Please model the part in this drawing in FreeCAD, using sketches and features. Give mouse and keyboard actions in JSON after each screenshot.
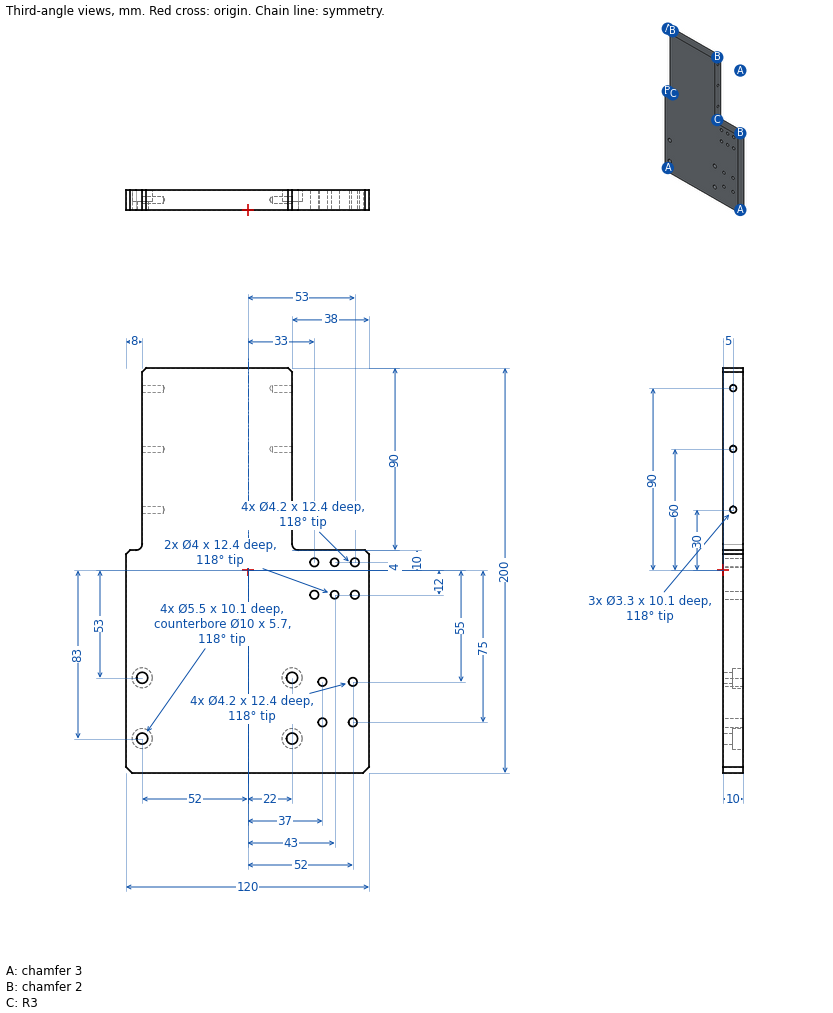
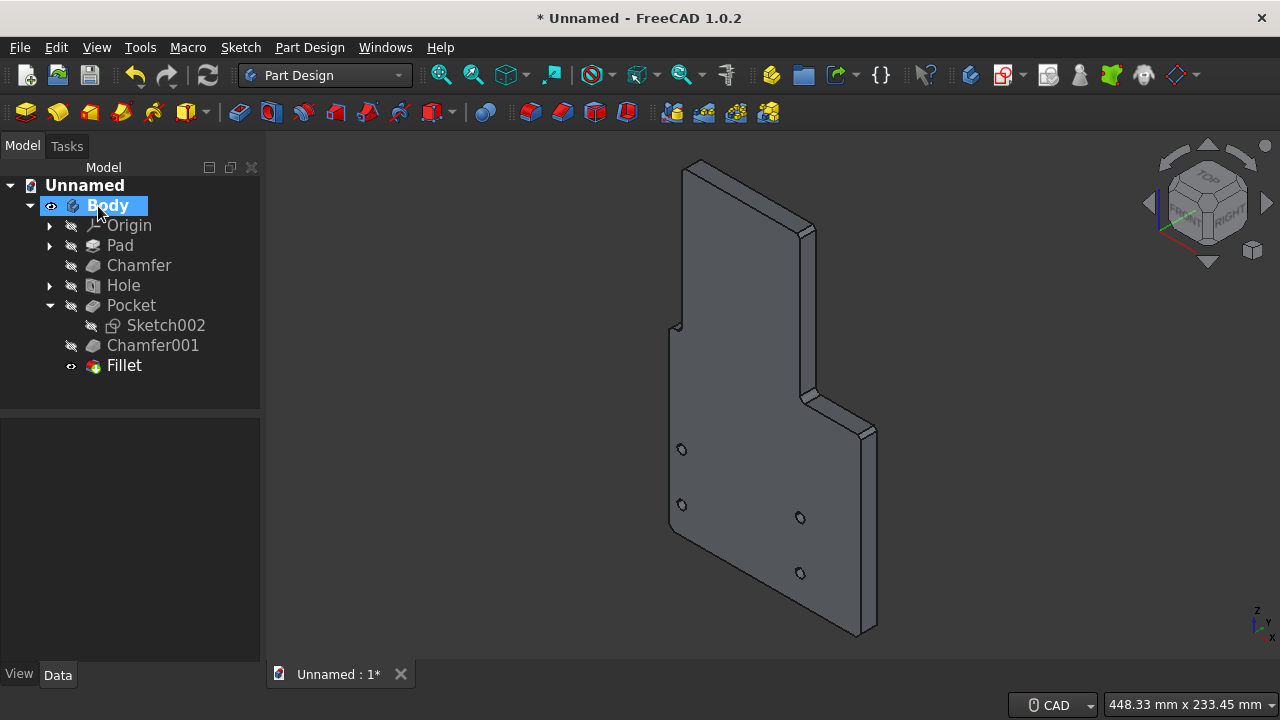
{"action": "key", "text": "6"}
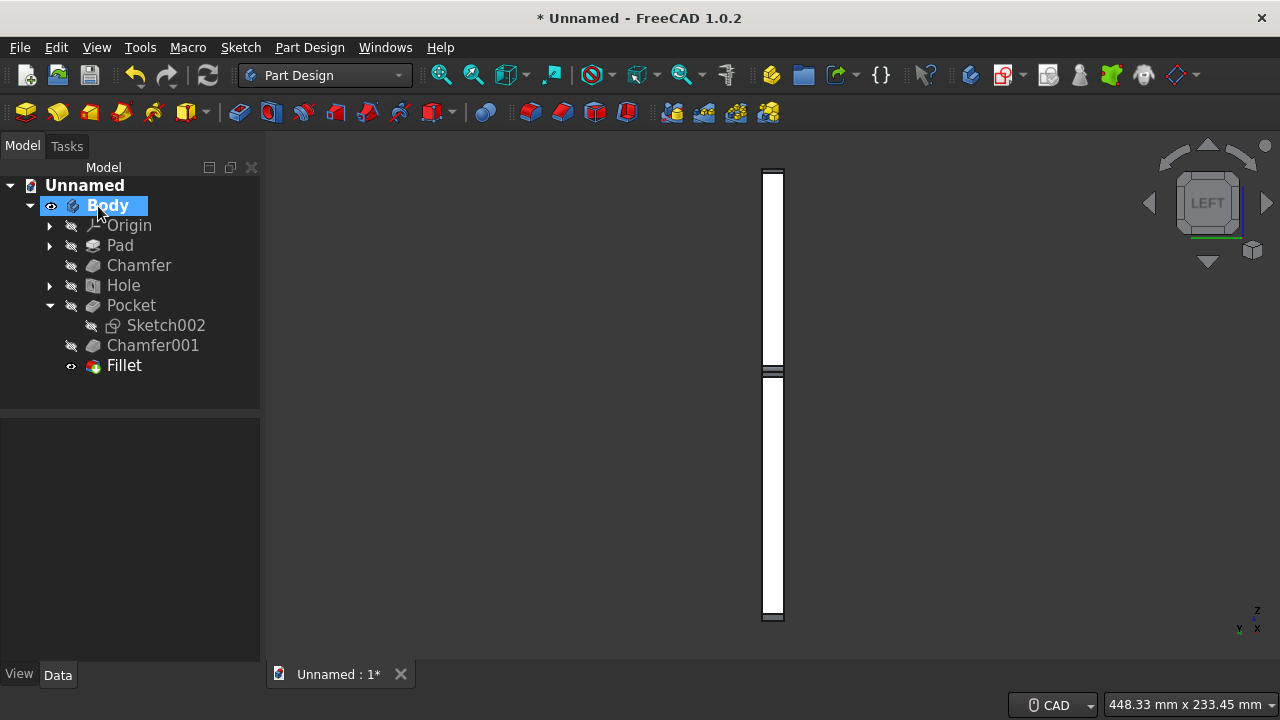
{"action": "left_click", "coordinate": [773, 323]}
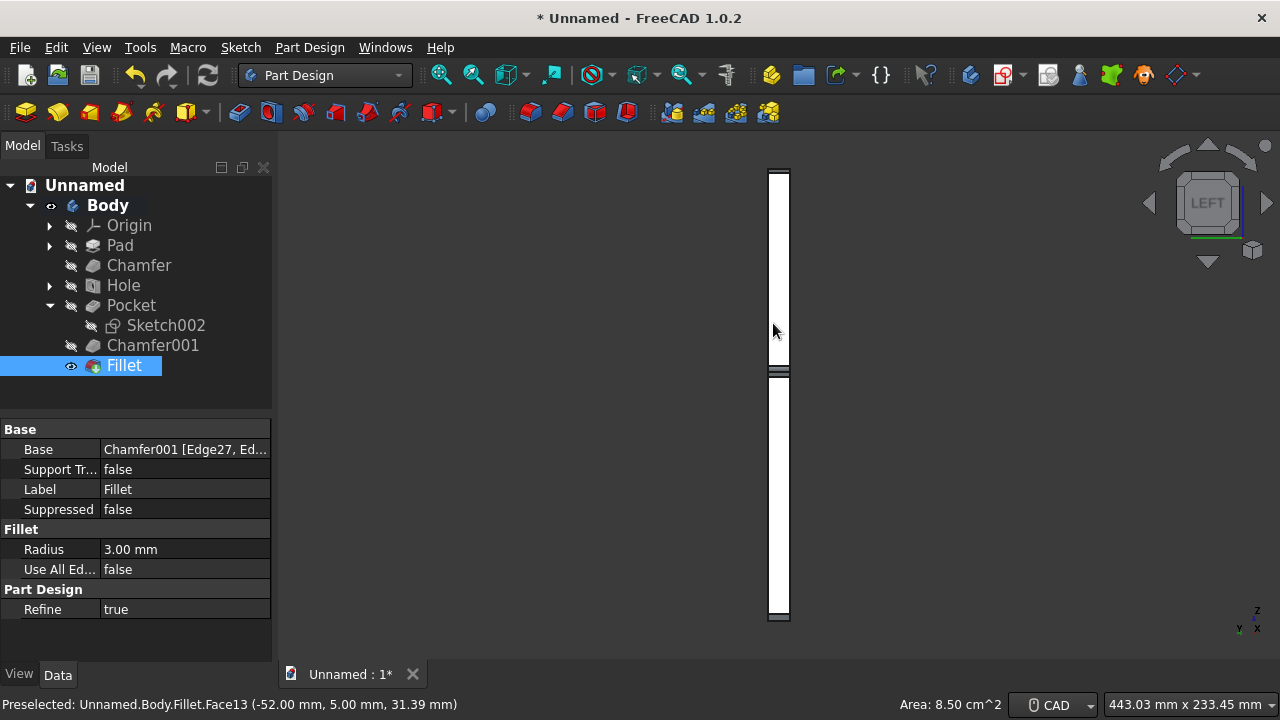
{"action": "left_click", "coordinate": [1004, 76]}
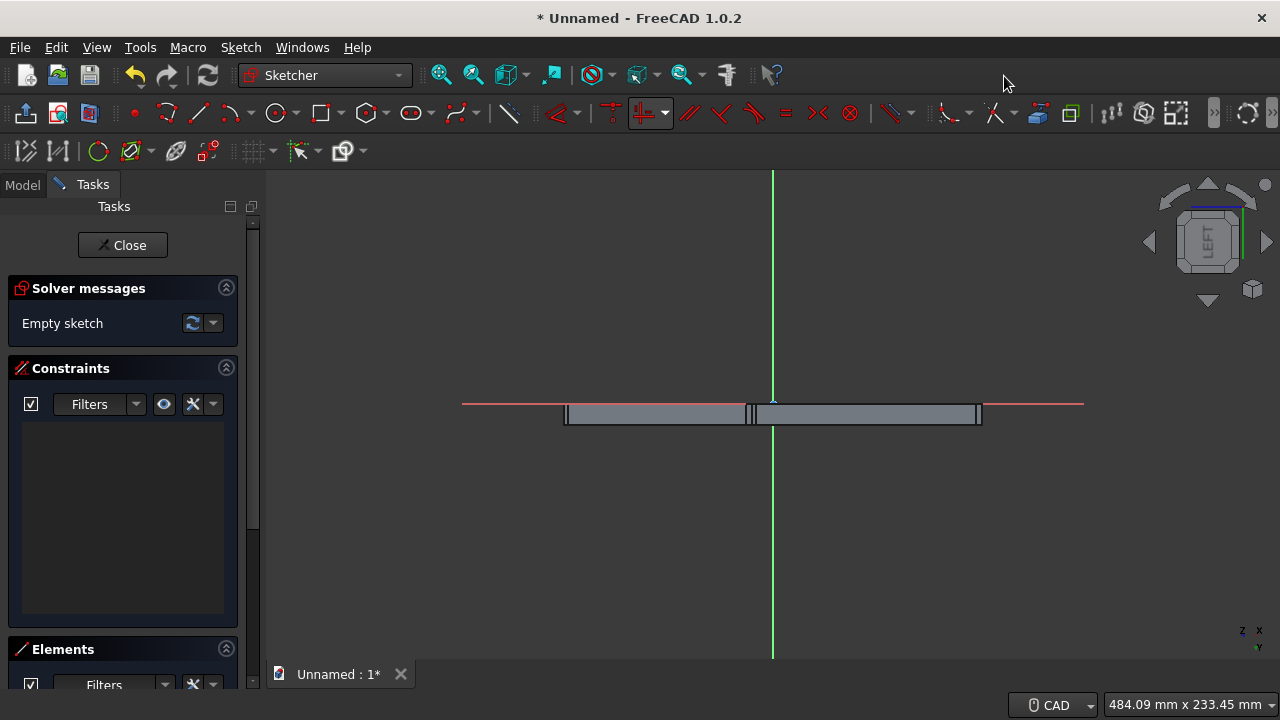
{"action": "left_click", "coordinate": [90, 114]}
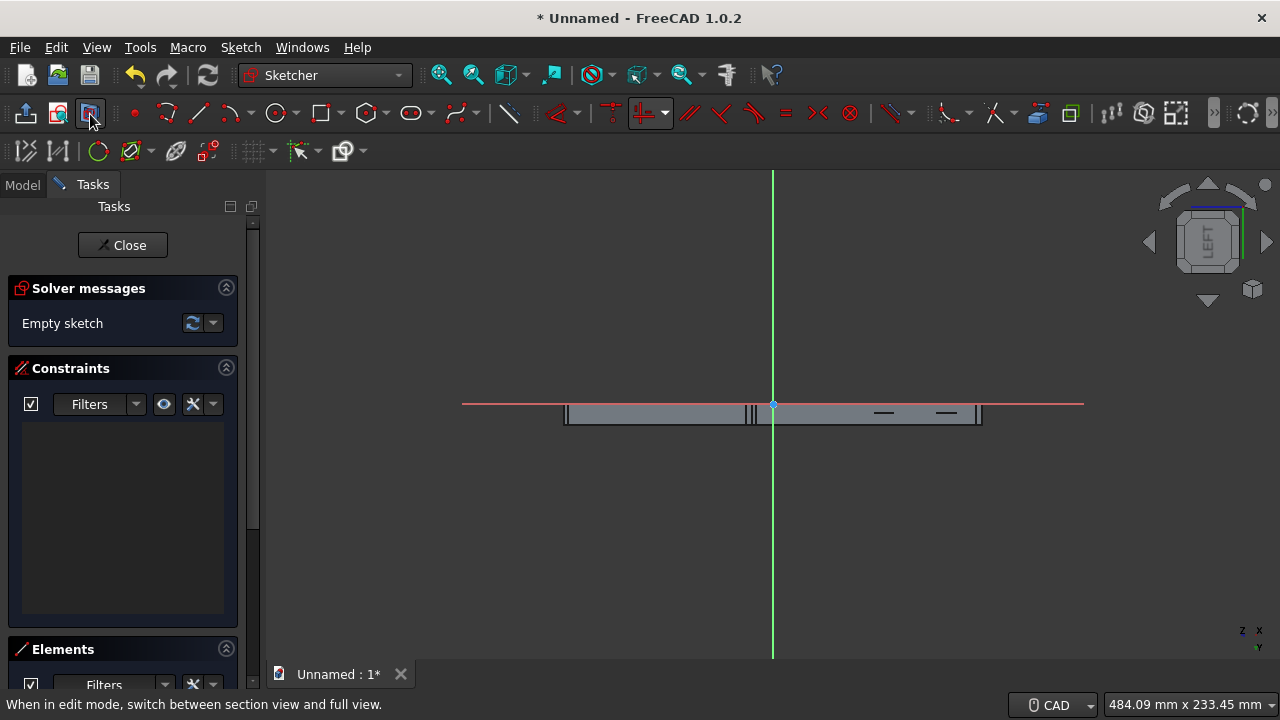
{"action": "scroll", "coordinate": [665, 409], "scroll_direction": "up", "scroll_amount": 6}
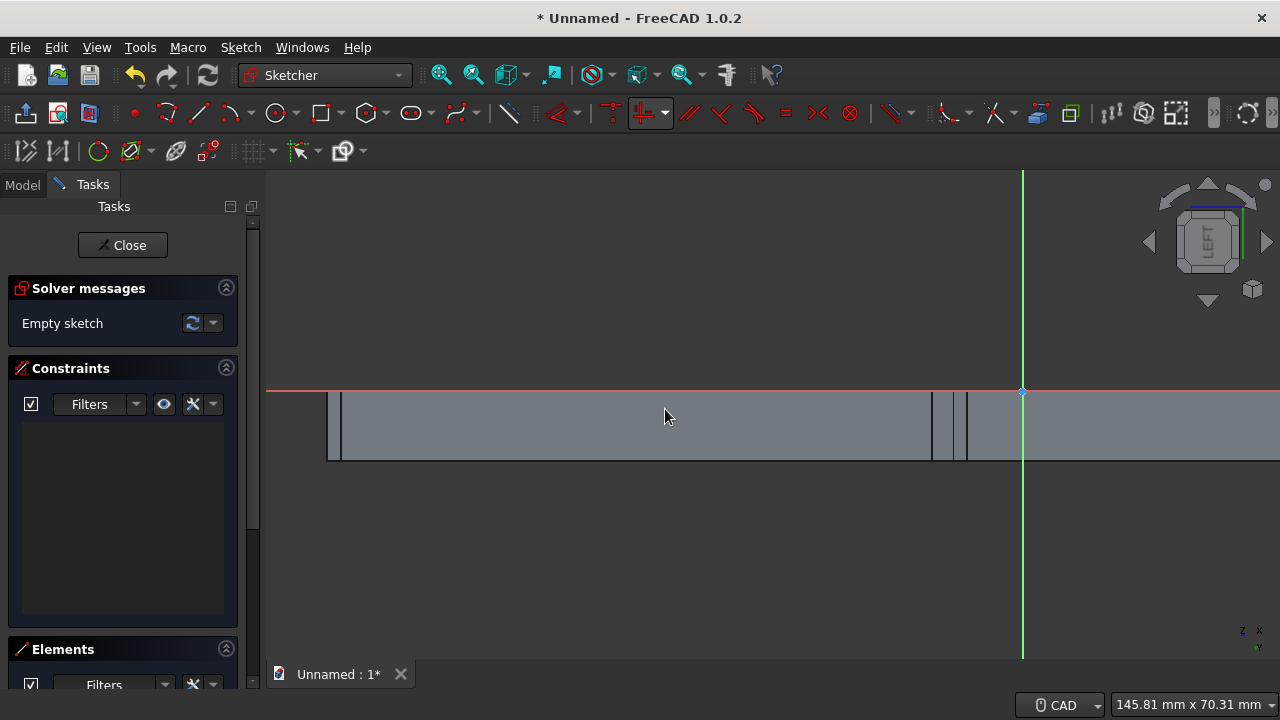
{"action": "key", "text": "g c"}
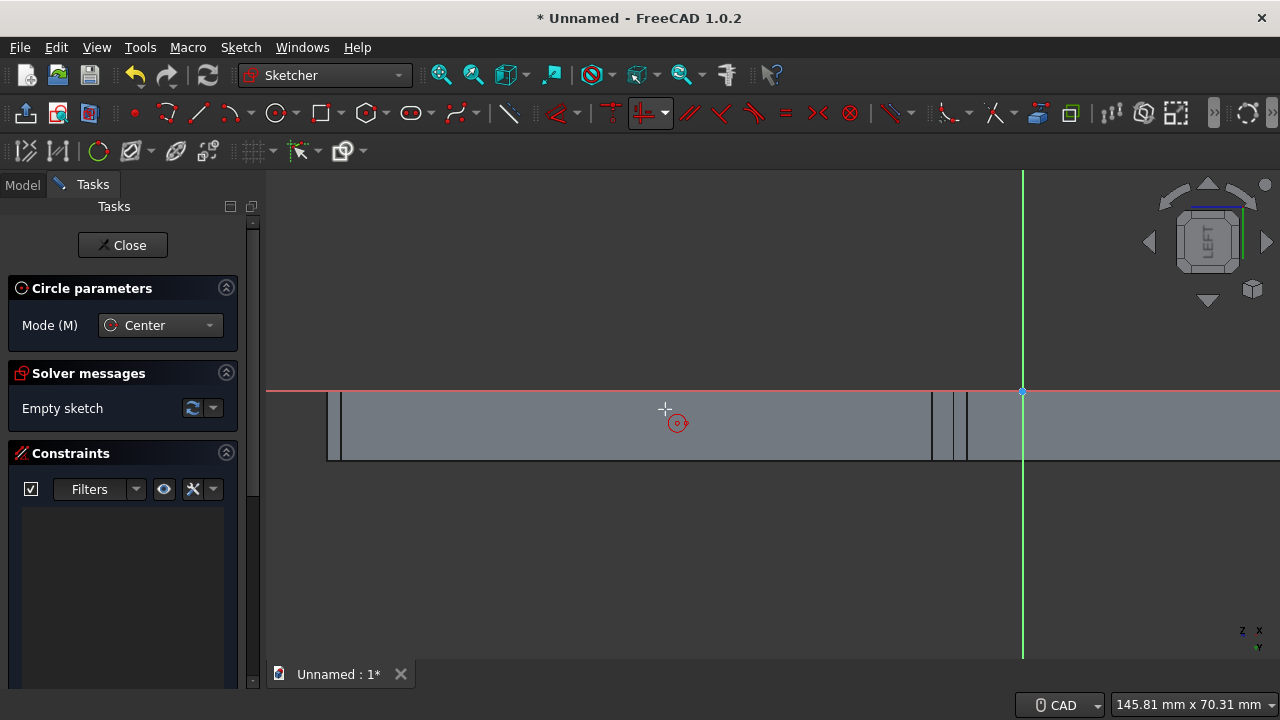
{"action": "scroll", "coordinate": [814, 426], "scroll_direction": "up", "scroll_amount": 4}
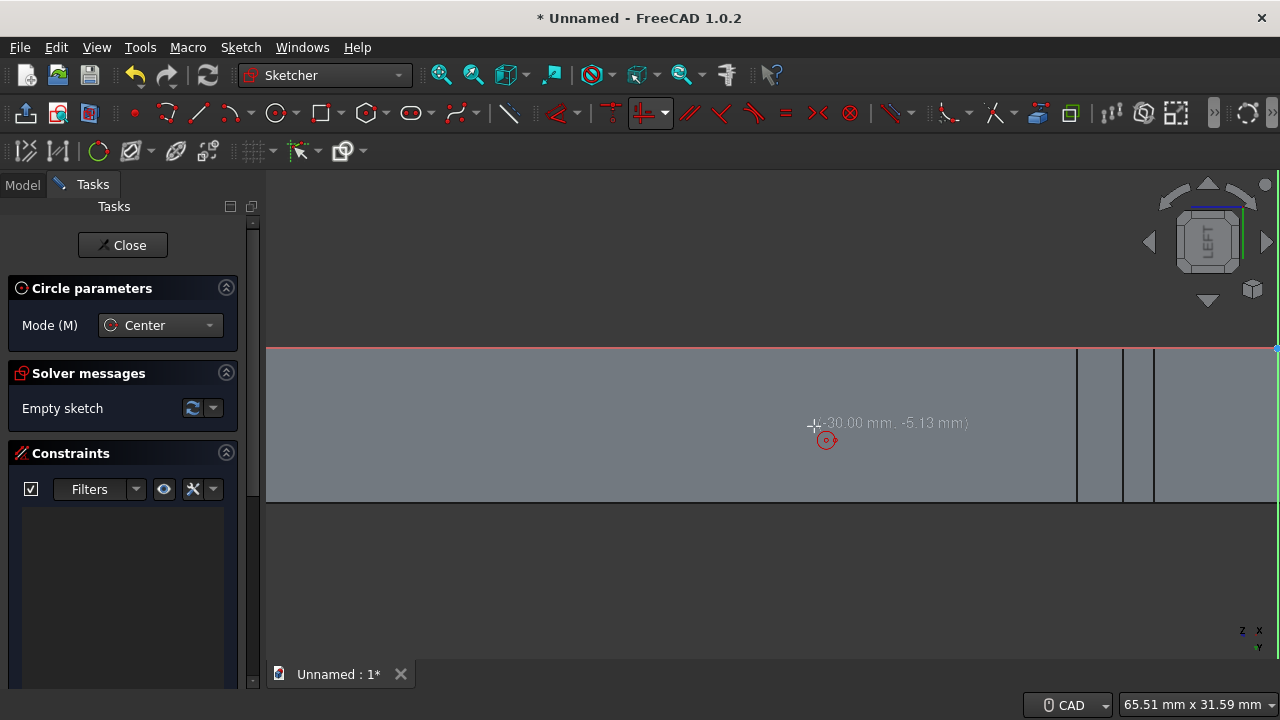
{"action": "left_click", "coordinate": [813, 426]}
{"action": "left_click", "coordinate": [831, 408]}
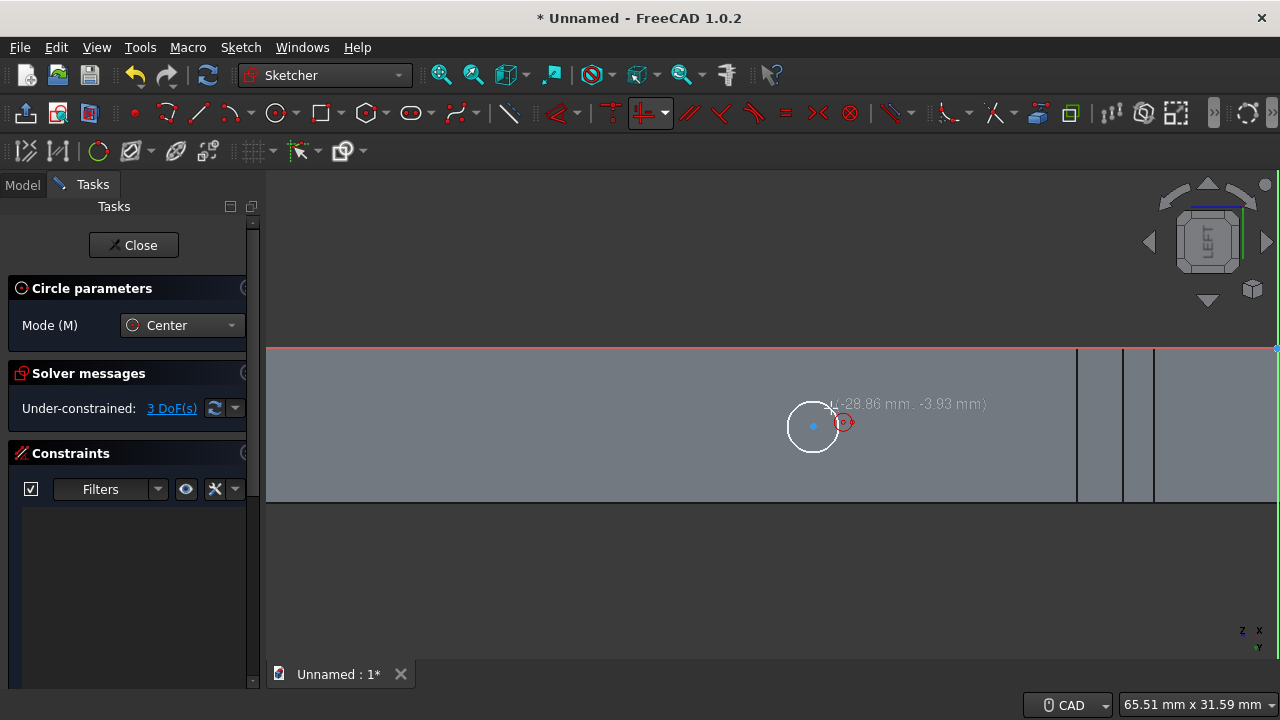
{"action": "left_click", "coordinate": [349, 426]}
{"action": "left_click", "coordinate": [367, 408]}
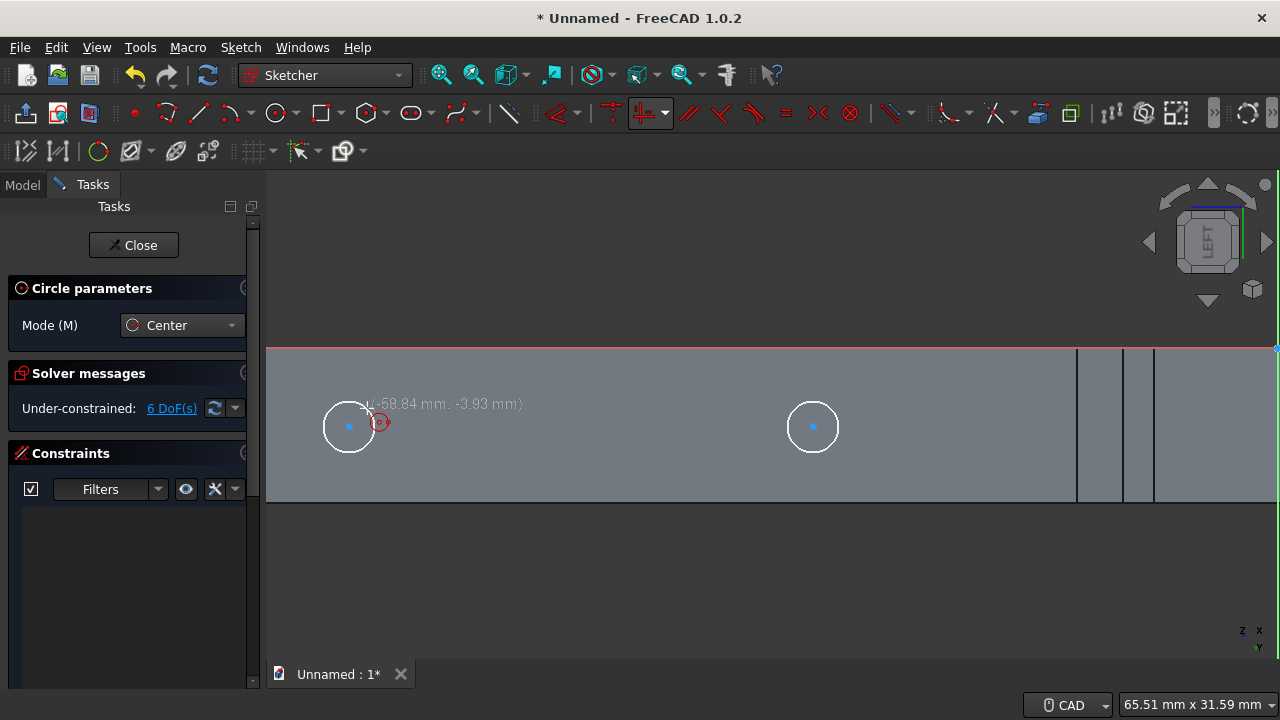
{"action": "scroll", "coordinate": [816, 427], "scroll_direction": "down", "scroll_amount": 4}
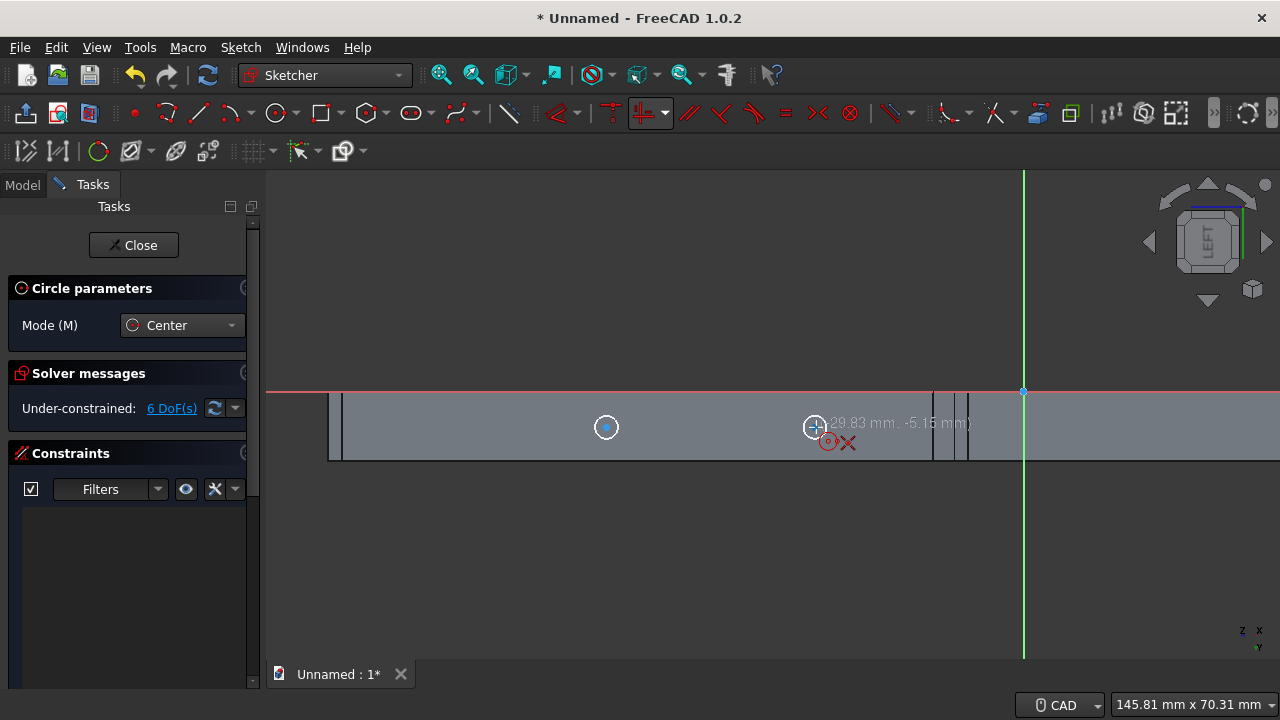
{"action": "scroll", "coordinate": [398, 427], "scroll_direction": "up", "scroll_amount": 4}